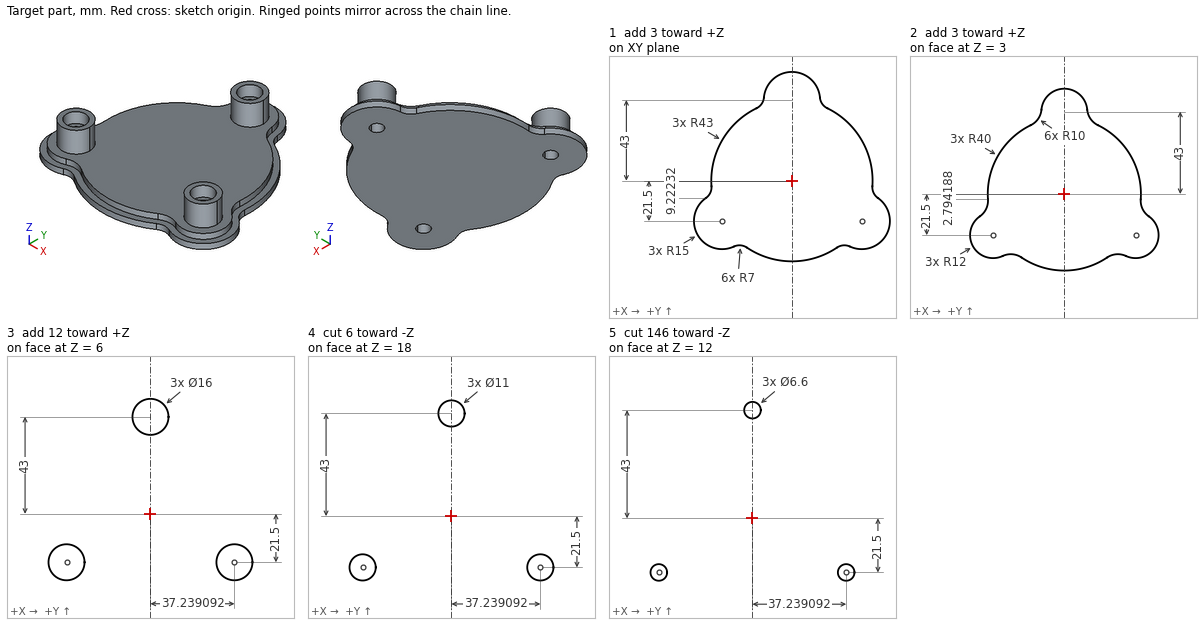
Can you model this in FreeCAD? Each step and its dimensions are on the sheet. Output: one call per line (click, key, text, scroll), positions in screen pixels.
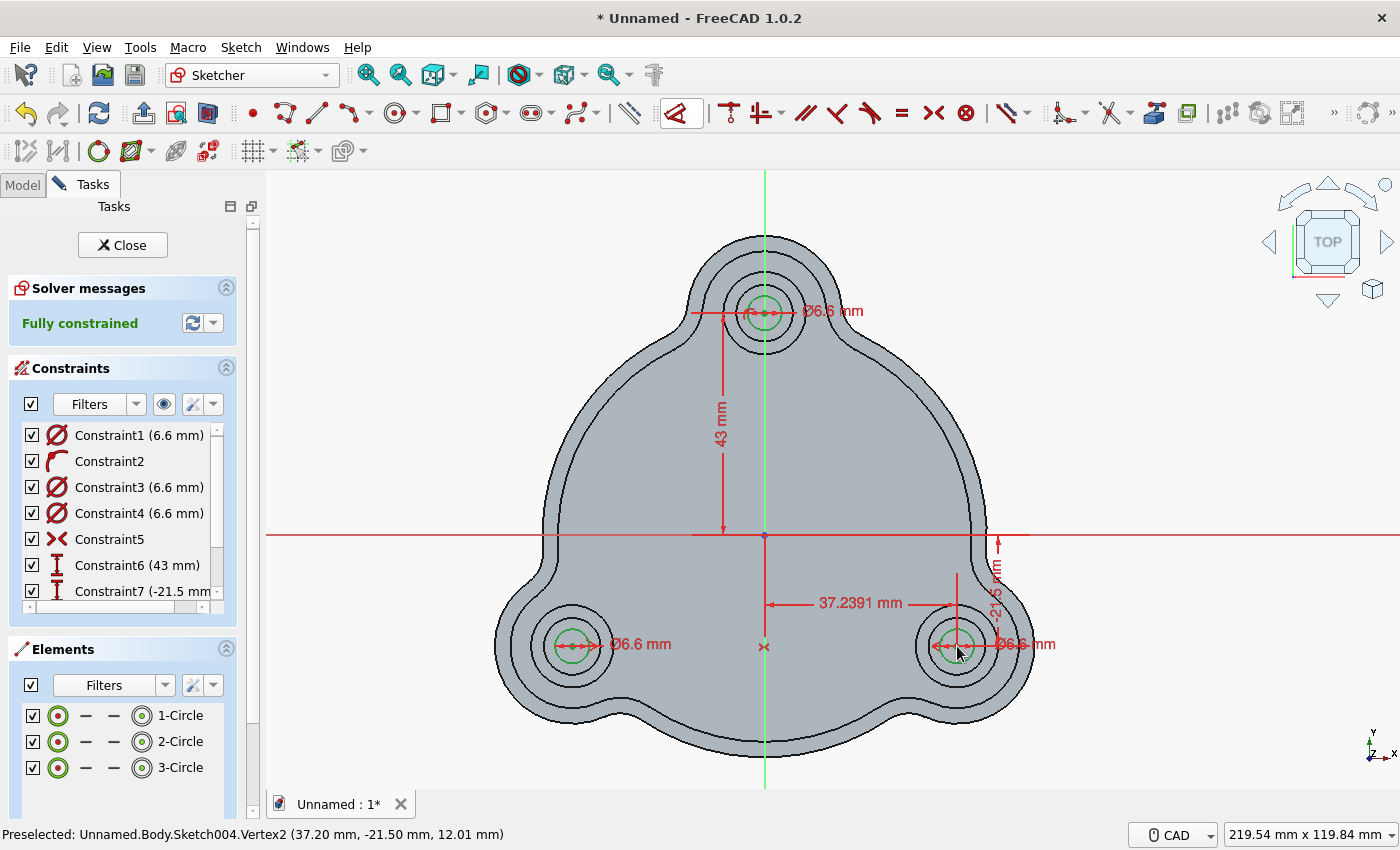
click(123, 245)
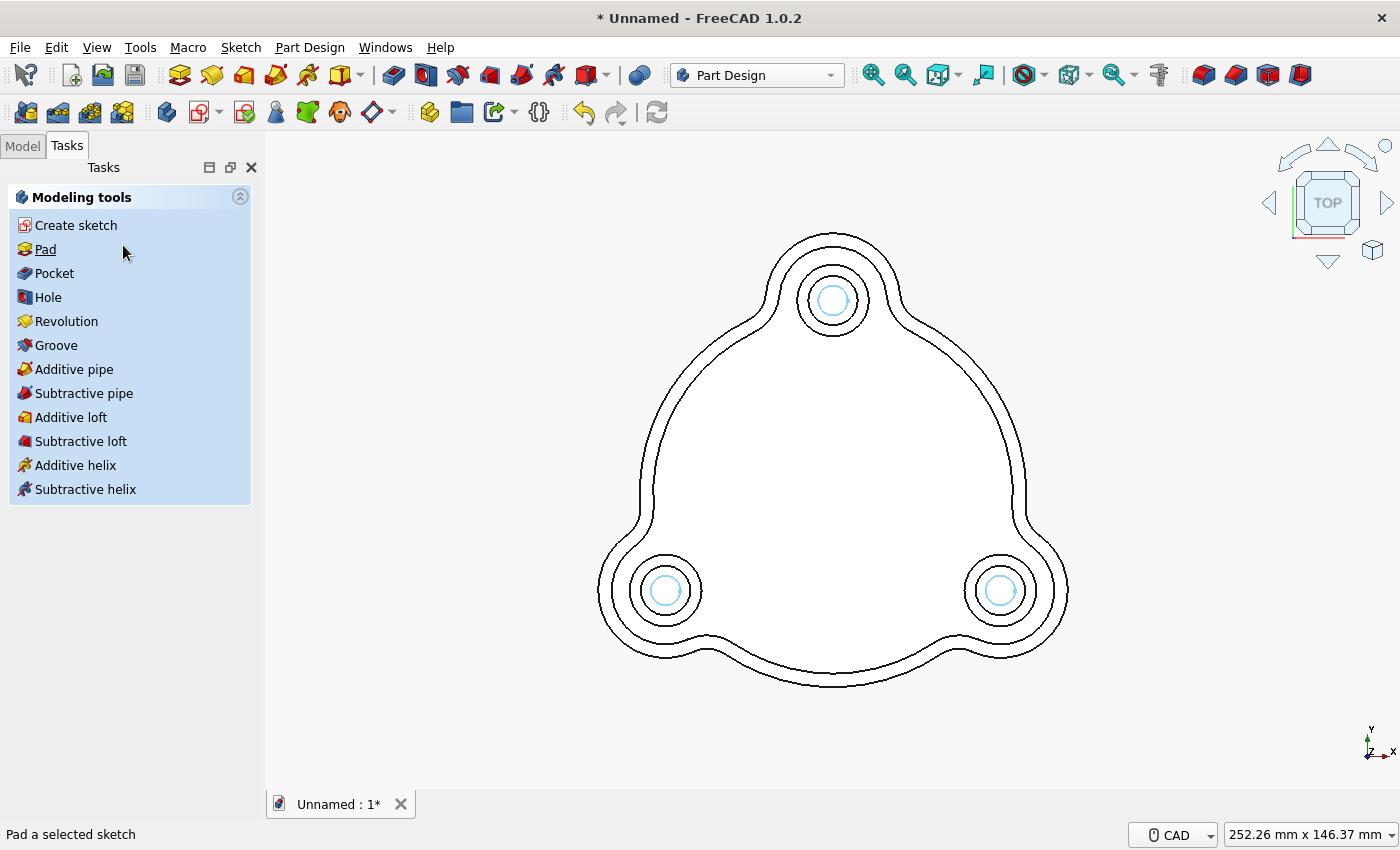
click(394, 76)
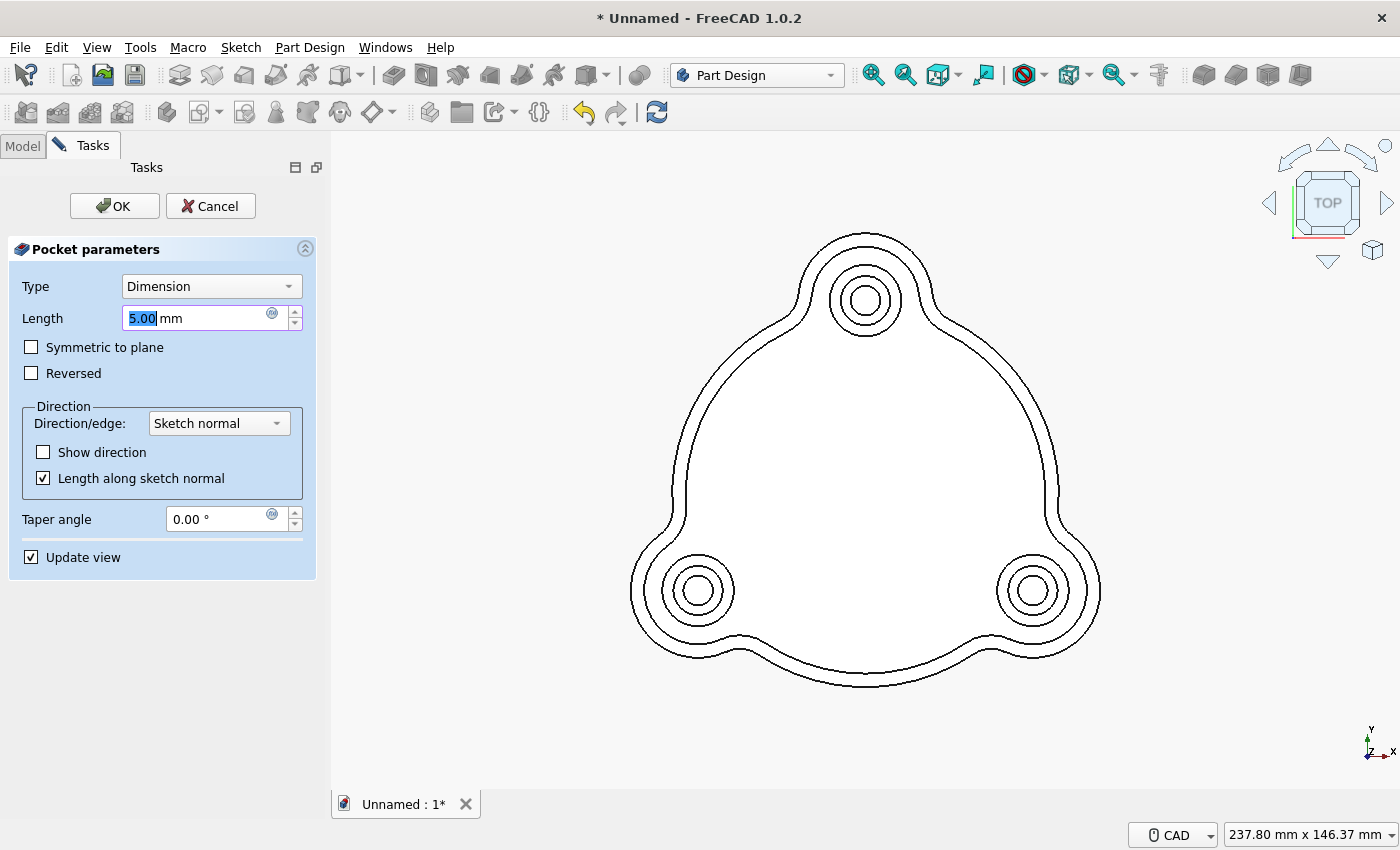
text(146)
key(Tab)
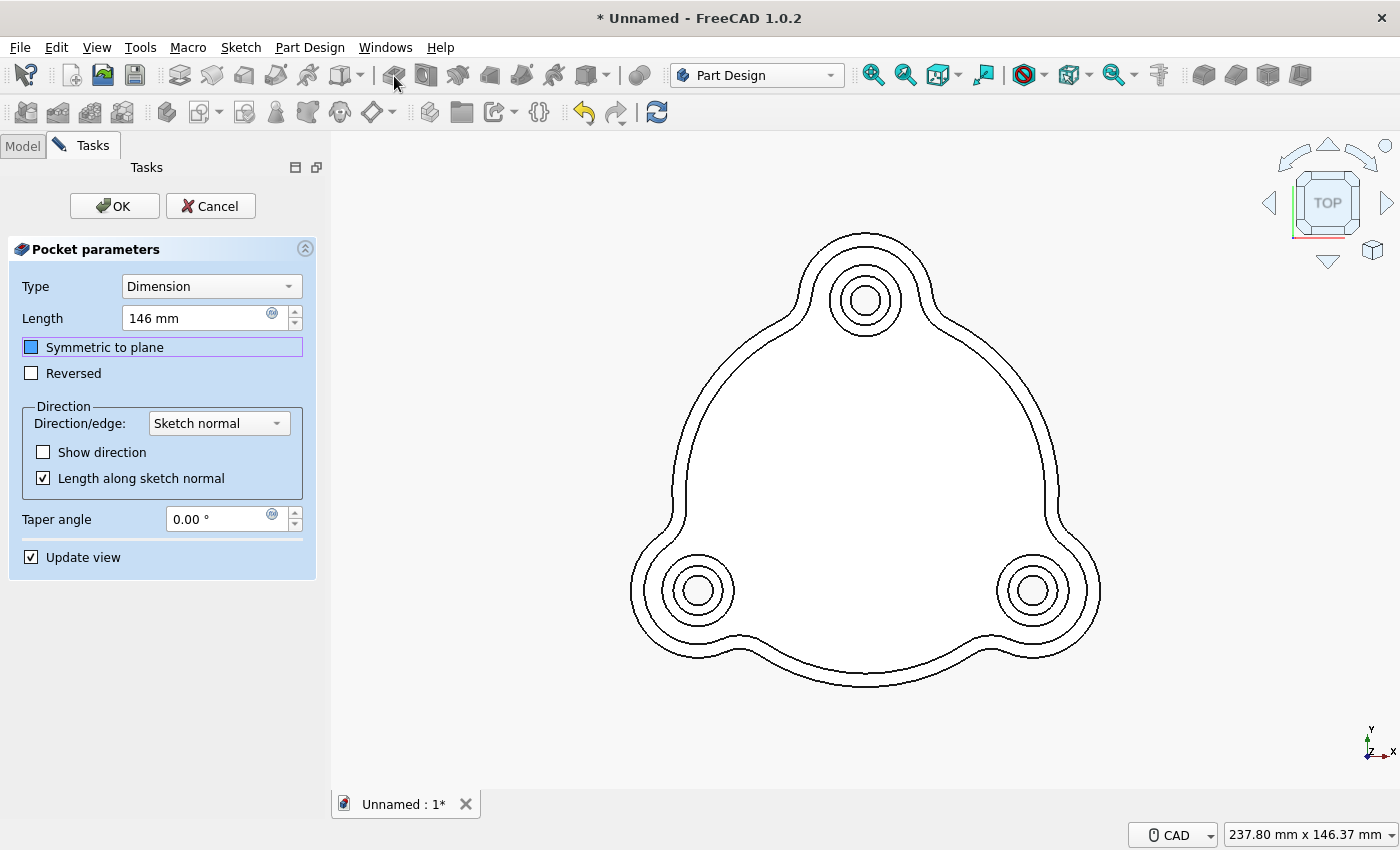
click(115, 206)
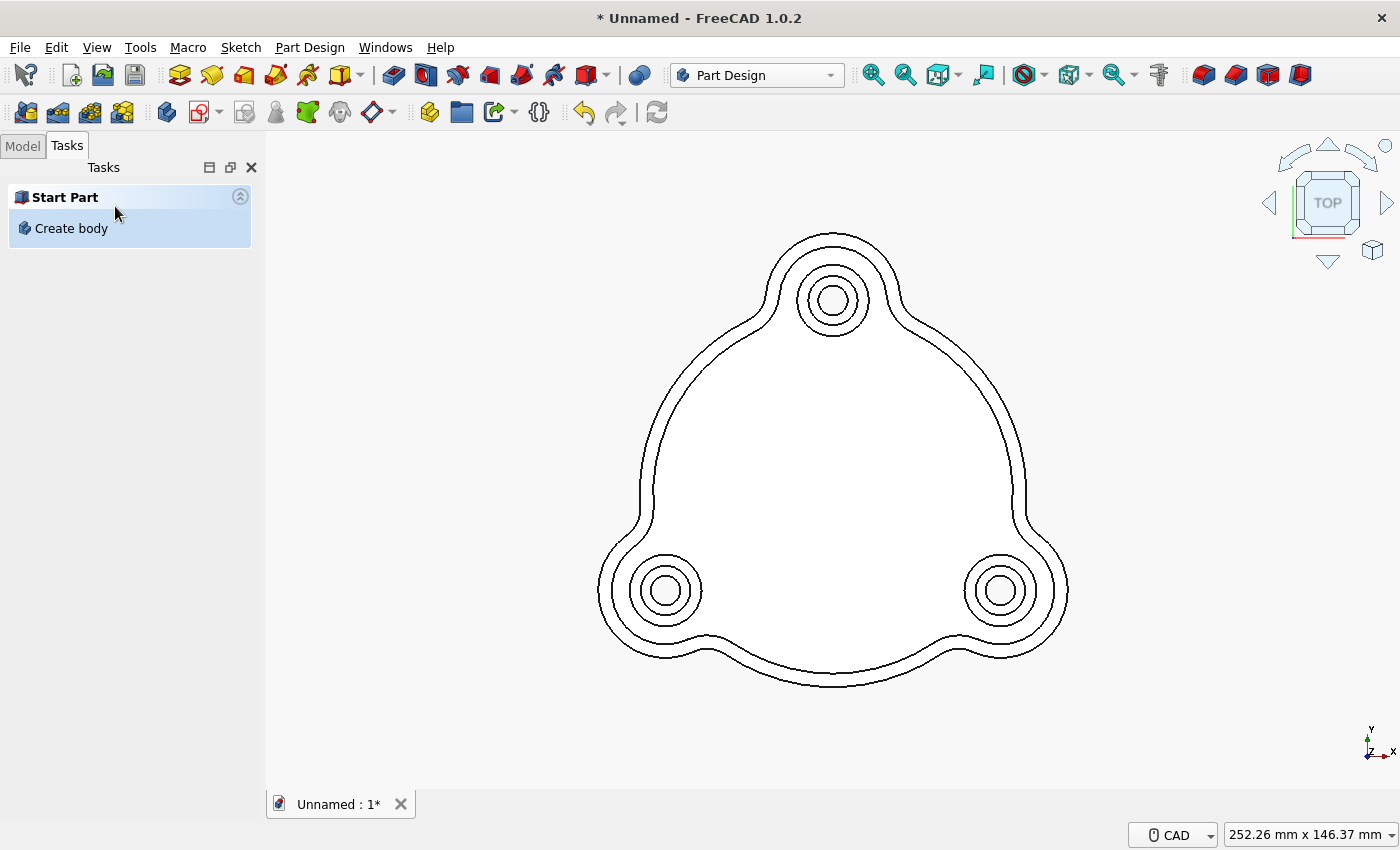
key(0)